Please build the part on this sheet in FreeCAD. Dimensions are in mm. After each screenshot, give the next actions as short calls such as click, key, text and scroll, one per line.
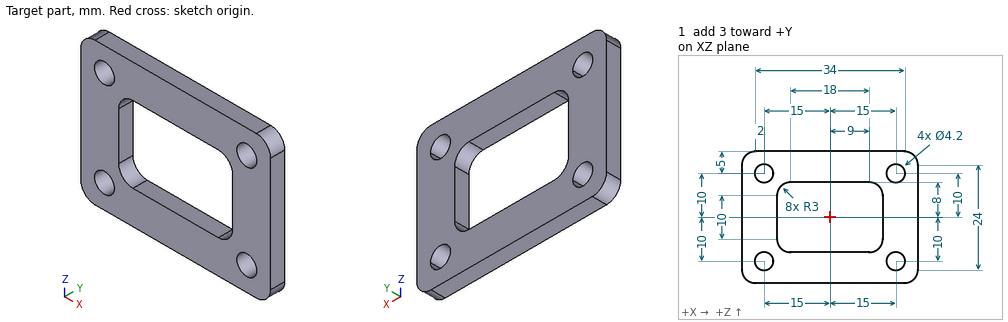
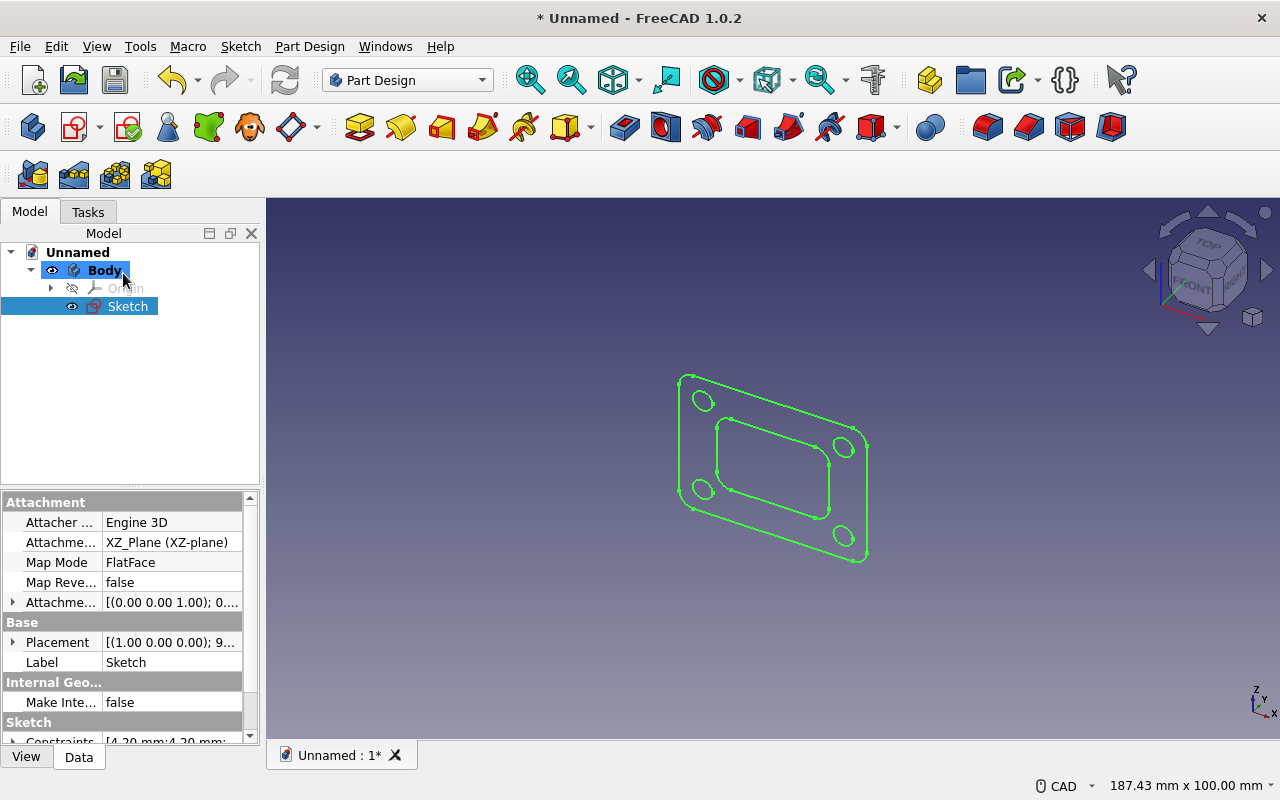
click(360, 128)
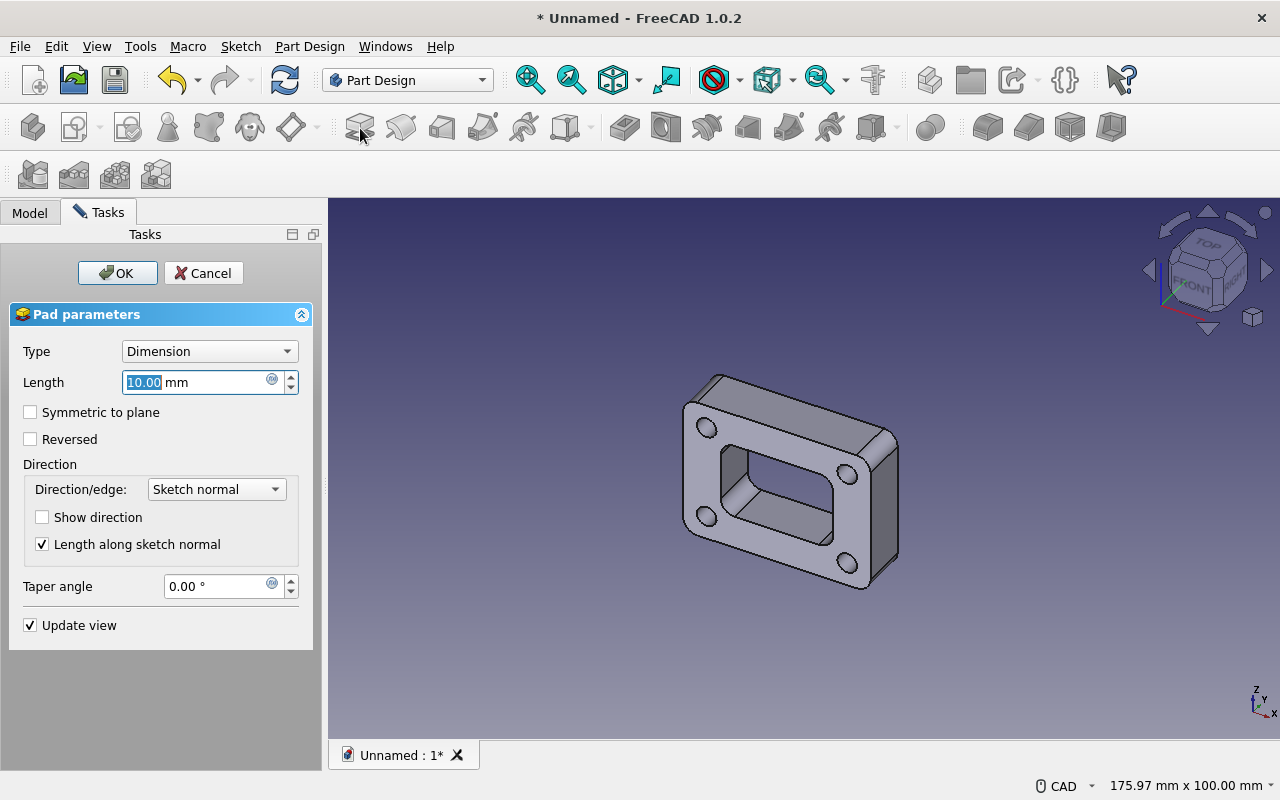
text(3)
key(Tab)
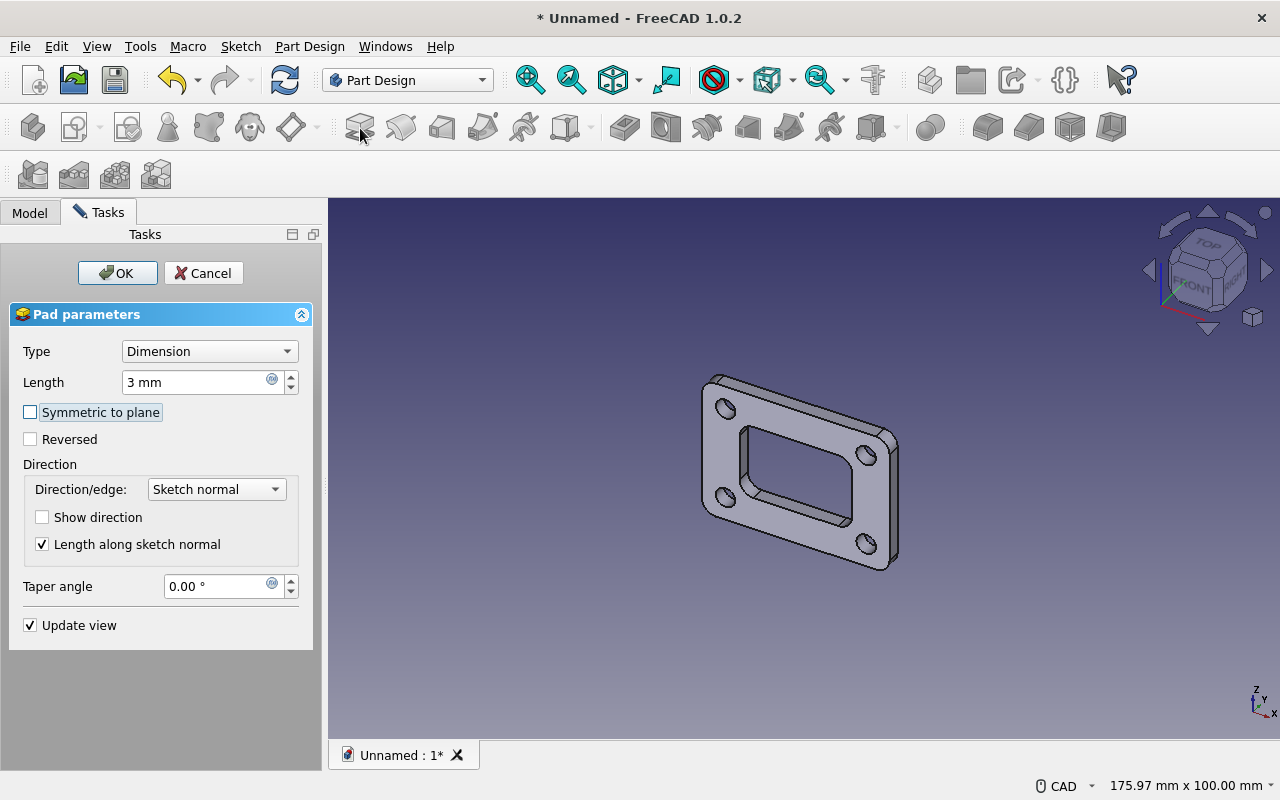
click(31, 439)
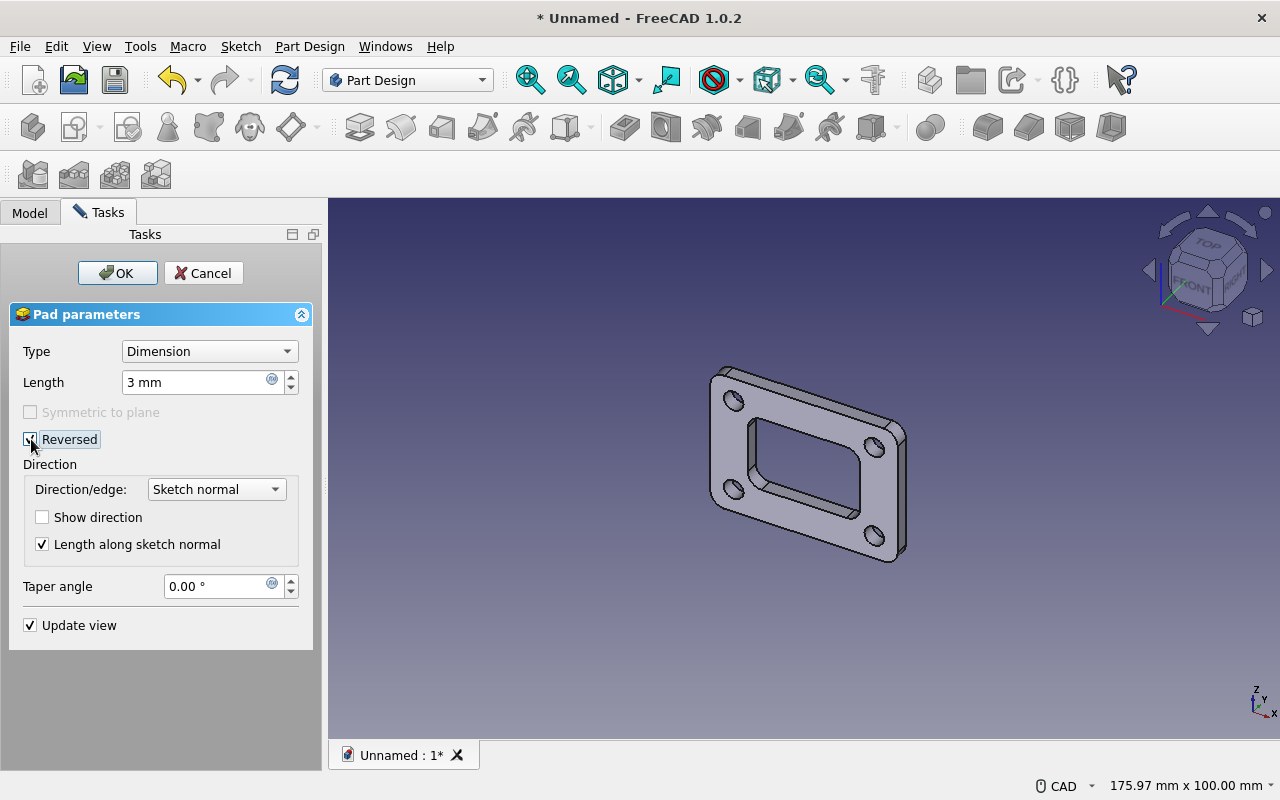
click(118, 273)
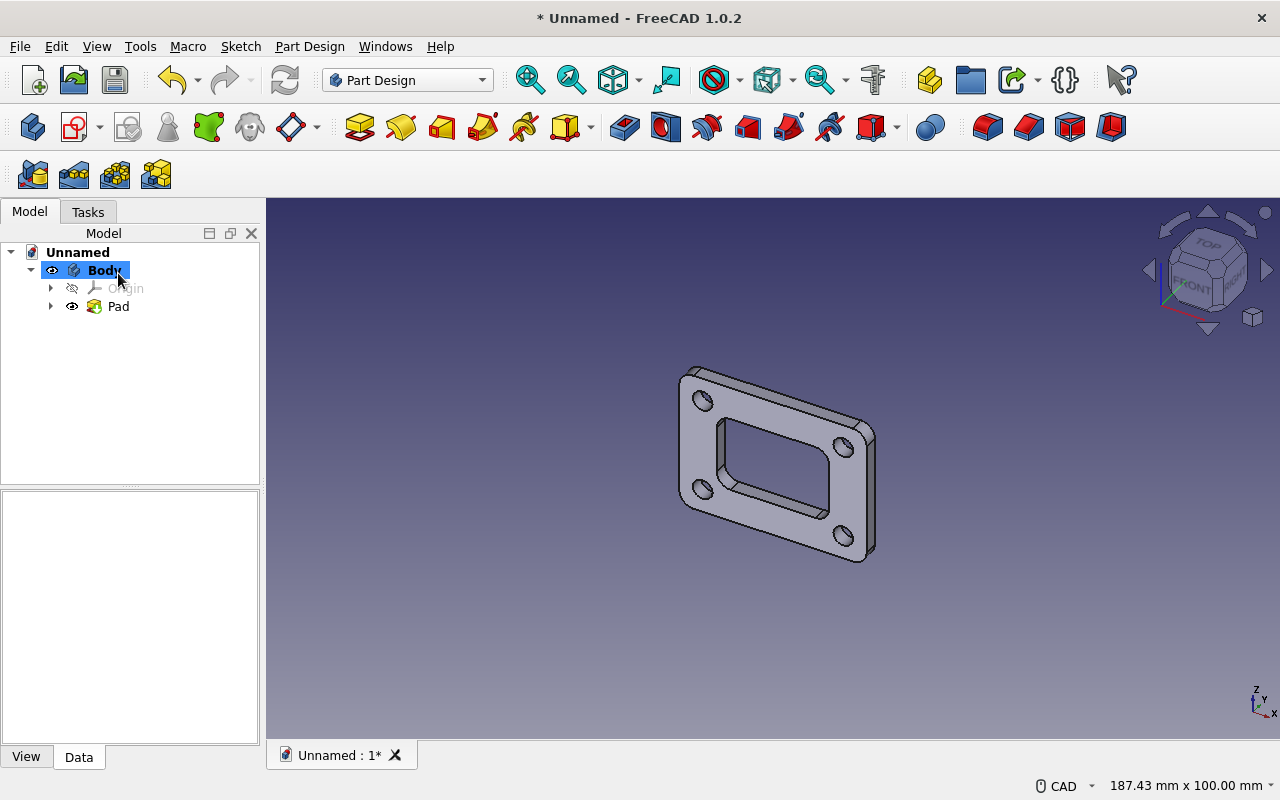
key(0)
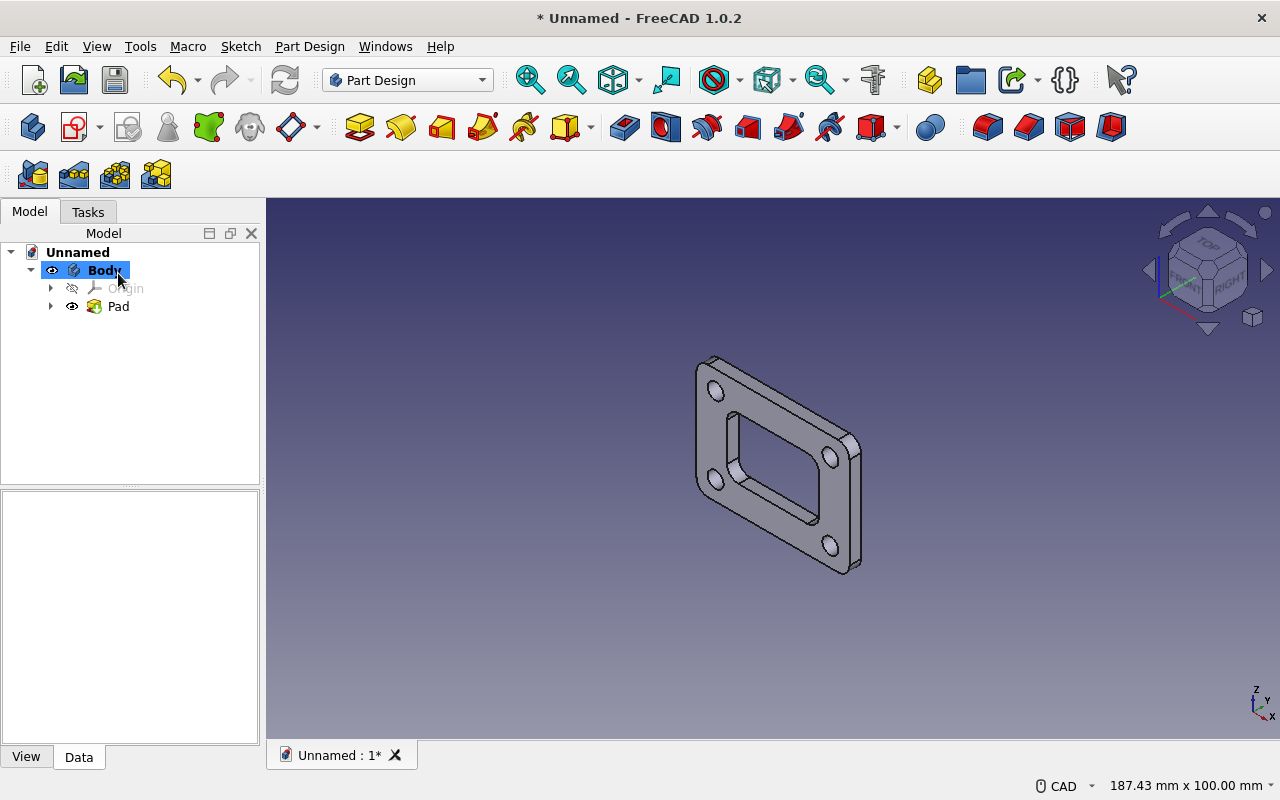
click(531, 80)